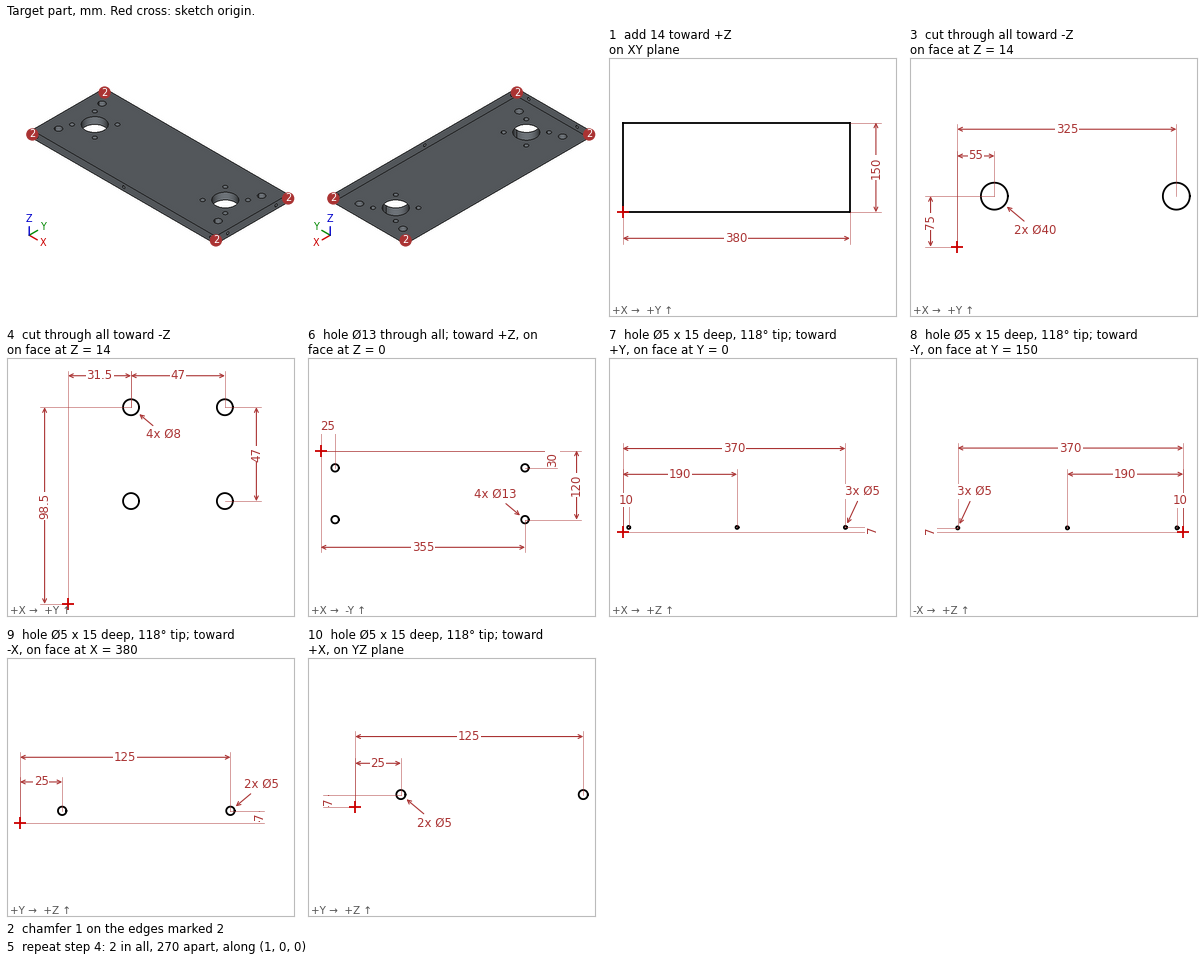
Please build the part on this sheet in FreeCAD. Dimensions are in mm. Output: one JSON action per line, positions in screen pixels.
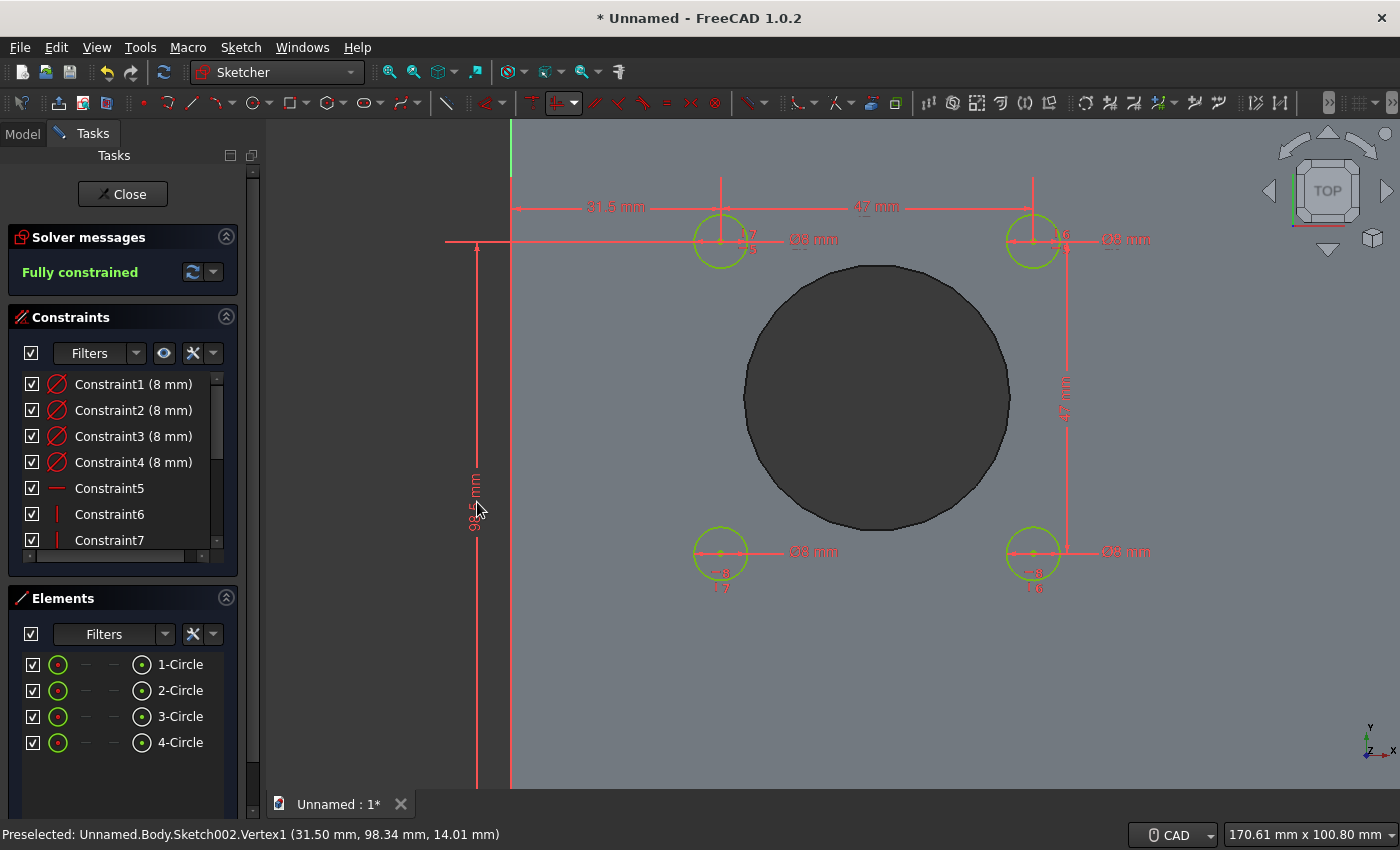
{"action": "left_click", "coordinate": [123, 194]}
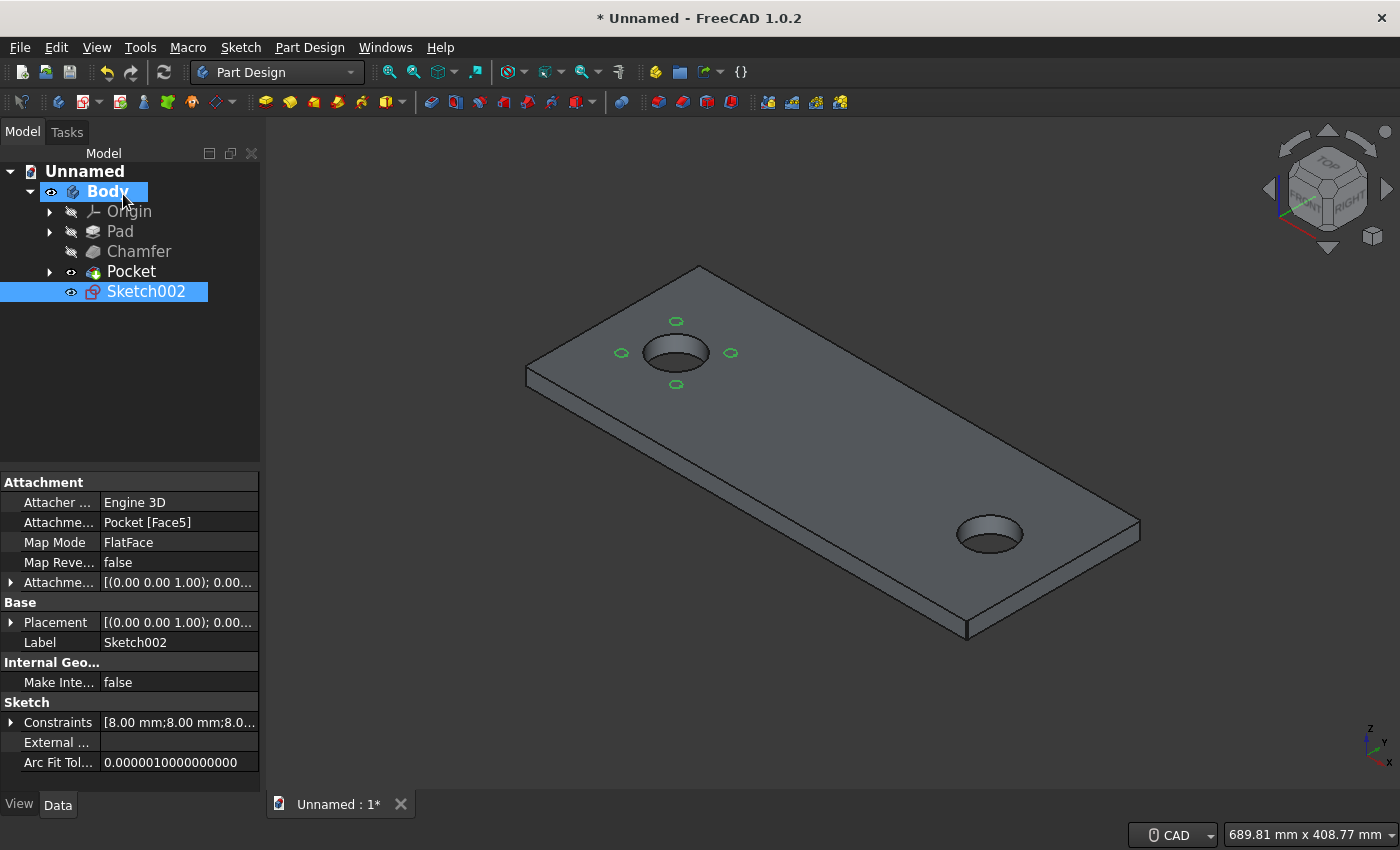
{"action": "left_click", "coordinate": [432, 102]}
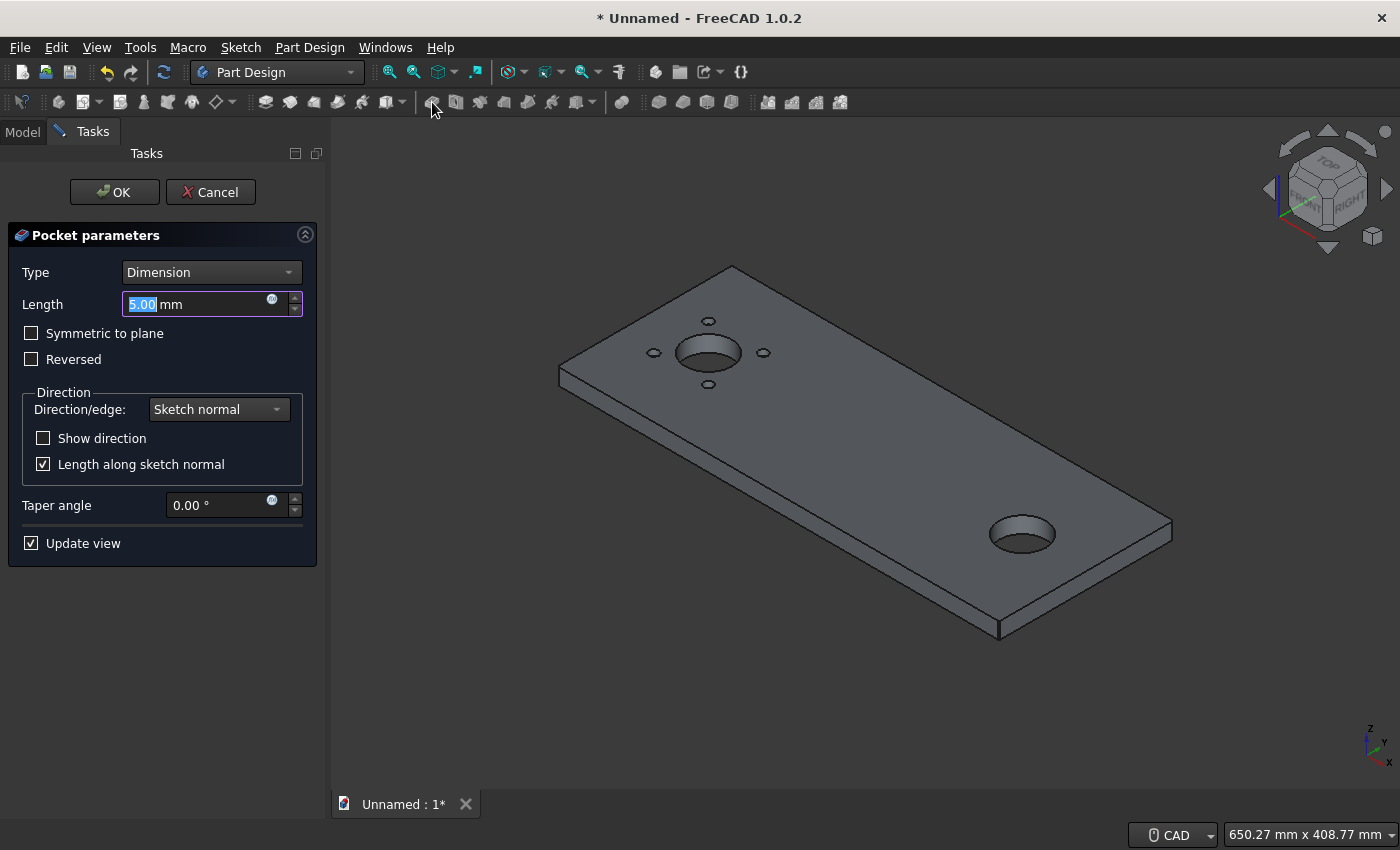
{"action": "left_click", "coordinate": [212, 272]}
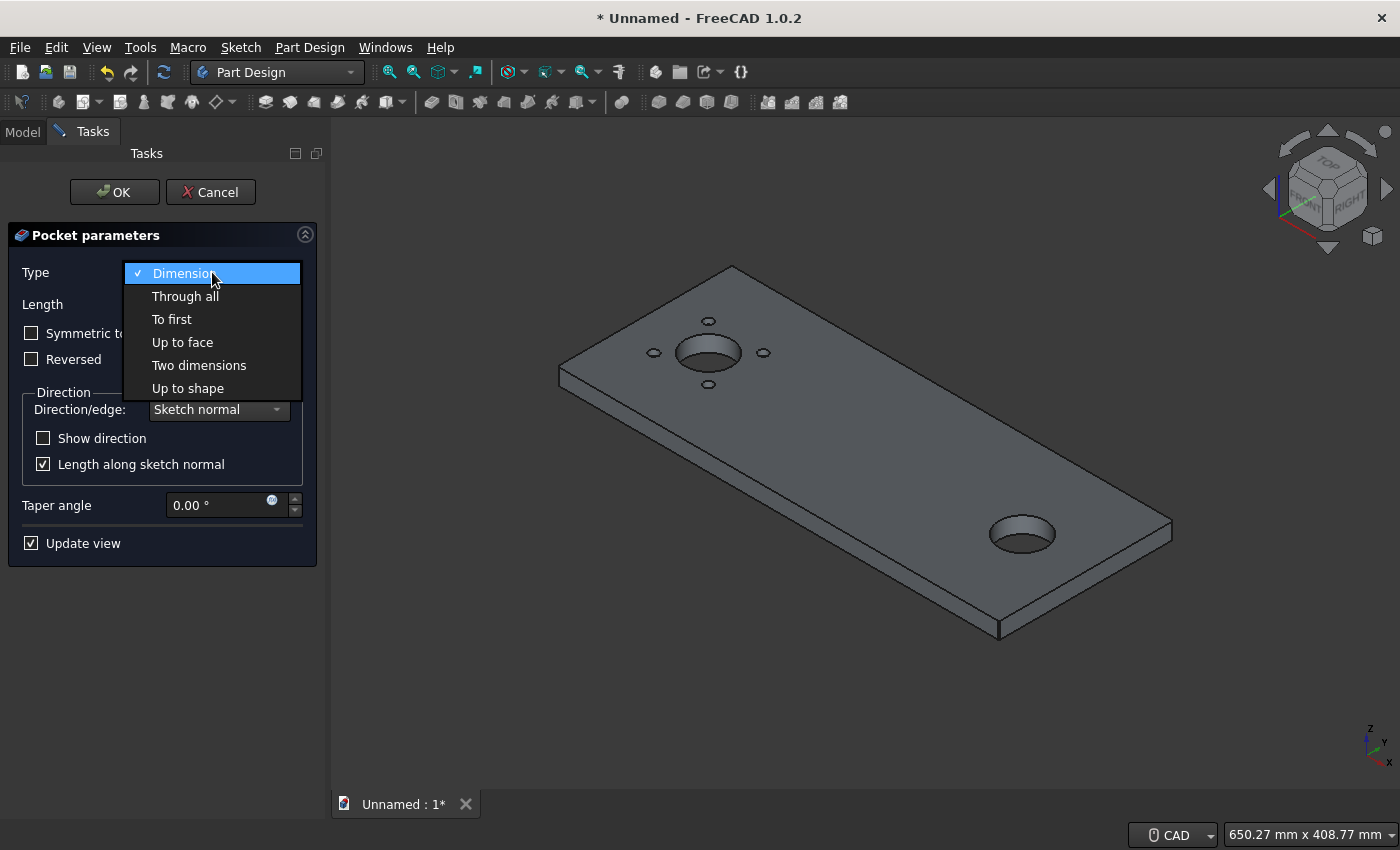
{"action": "left_click", "coordinate": [212, 296]}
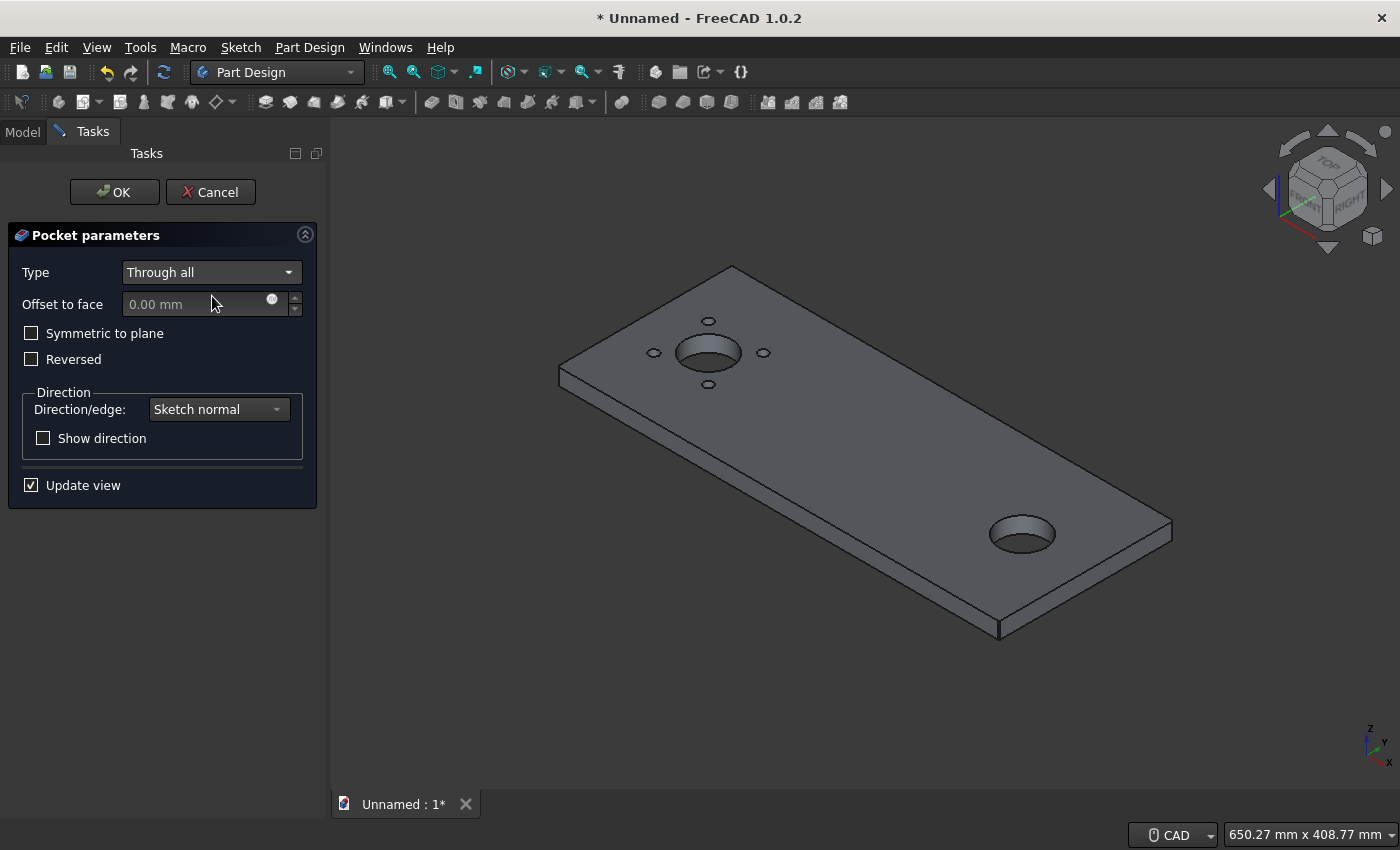
{"action": "left_click", "coordinate": [115, 192]}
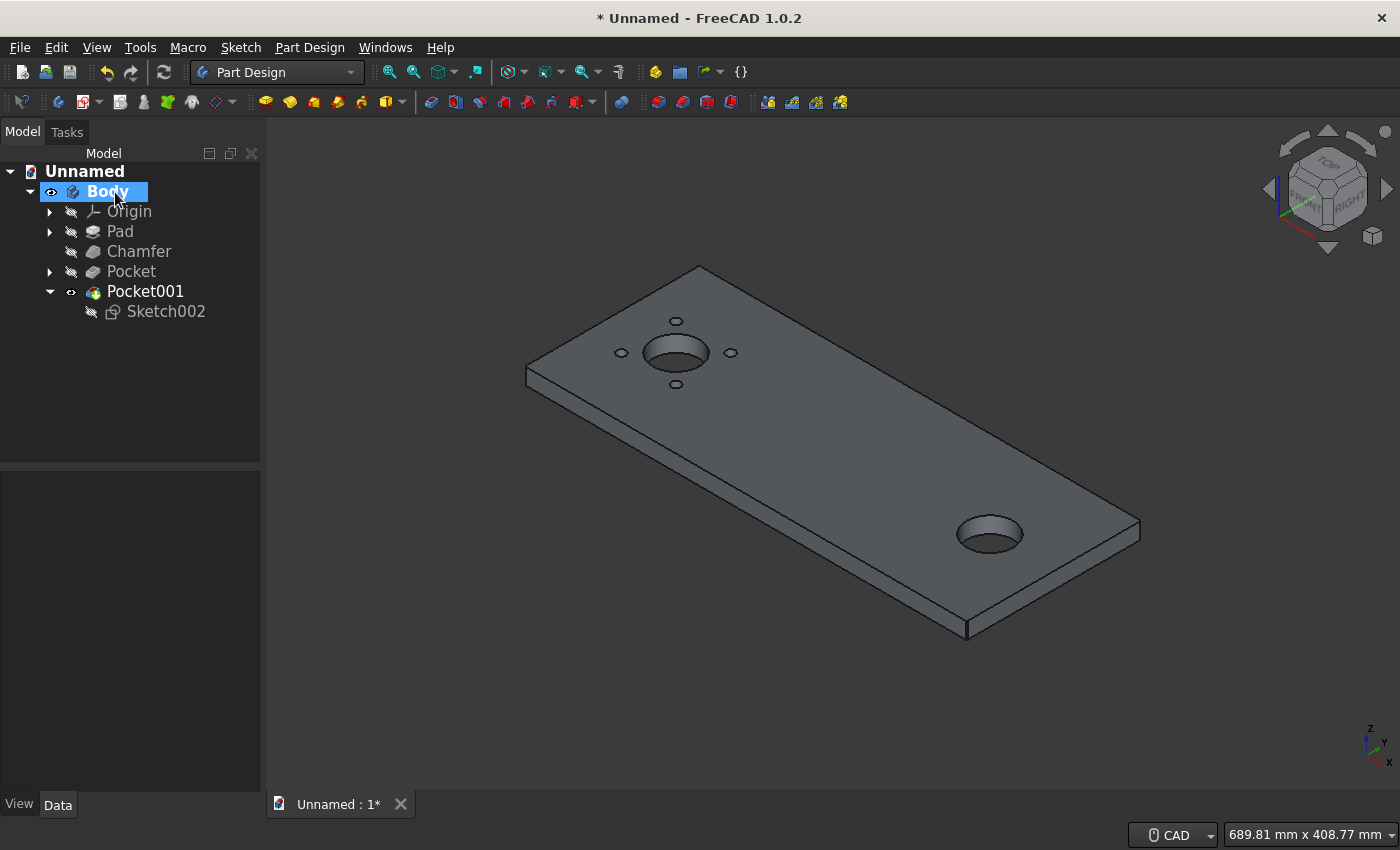
{"action": "left_click", "coordinate": [116, 292]}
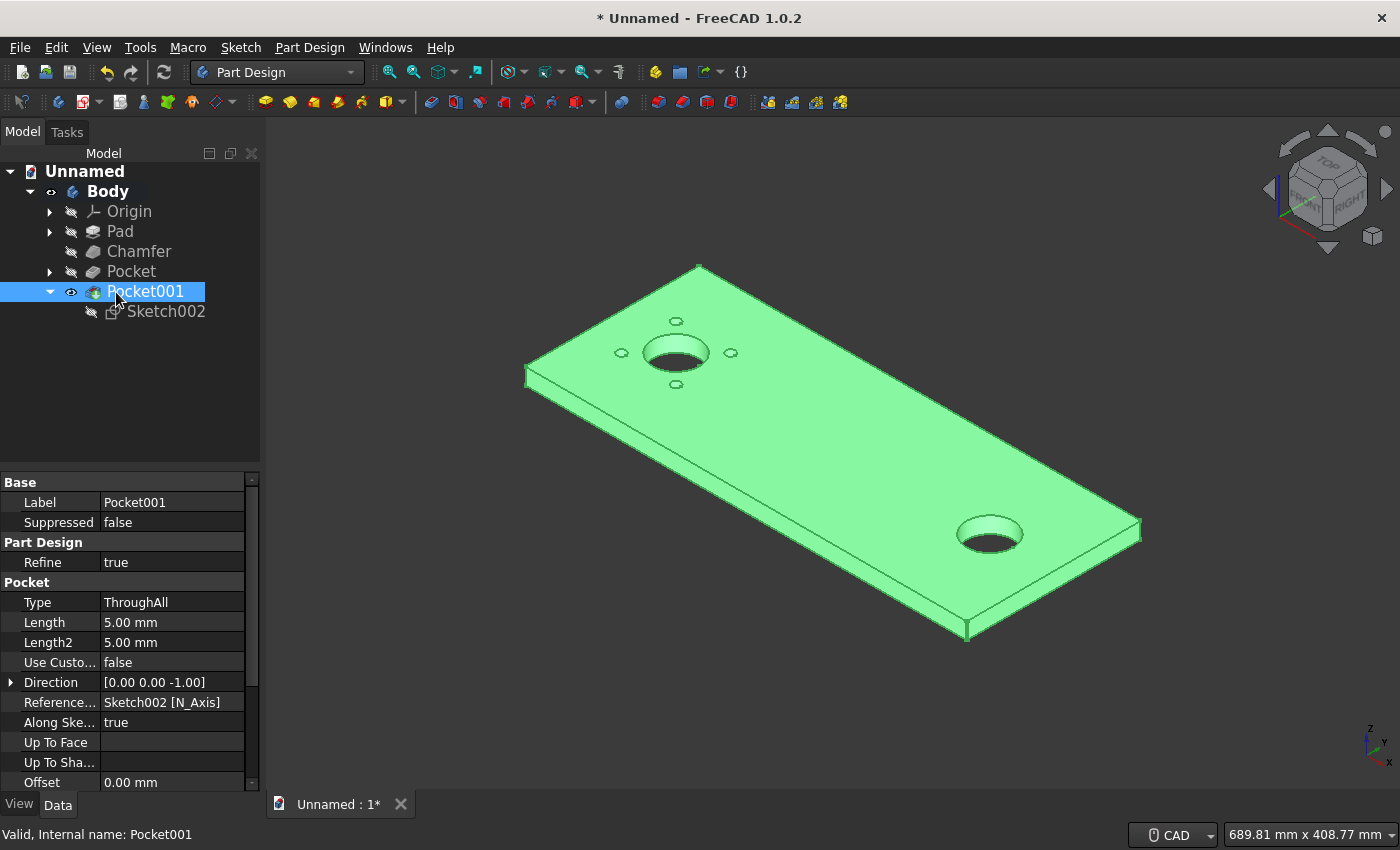
{"action": "left_click", "coordinate": [792, 102]}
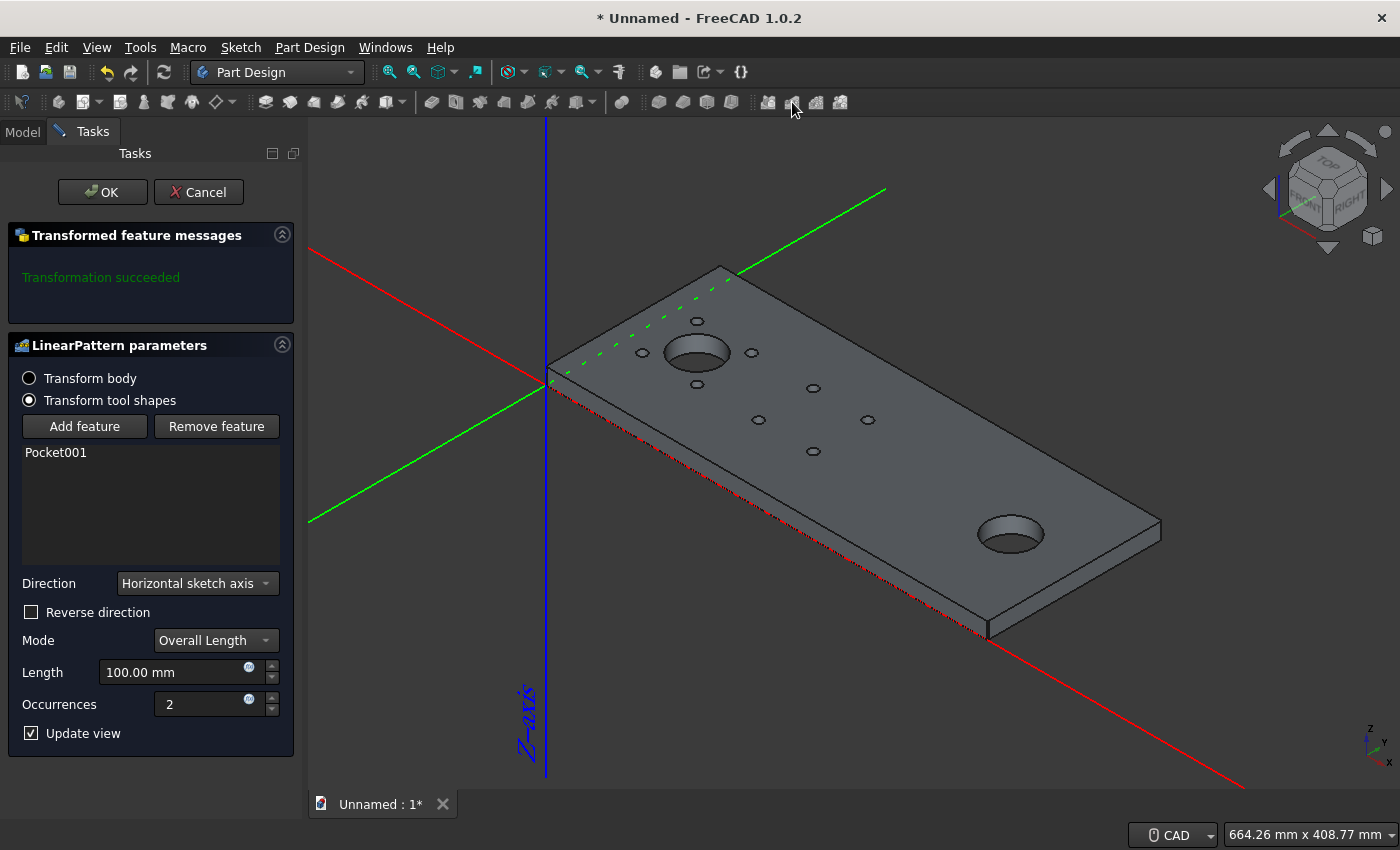
{"action": "left_click", "coordinate": [198, 584]}